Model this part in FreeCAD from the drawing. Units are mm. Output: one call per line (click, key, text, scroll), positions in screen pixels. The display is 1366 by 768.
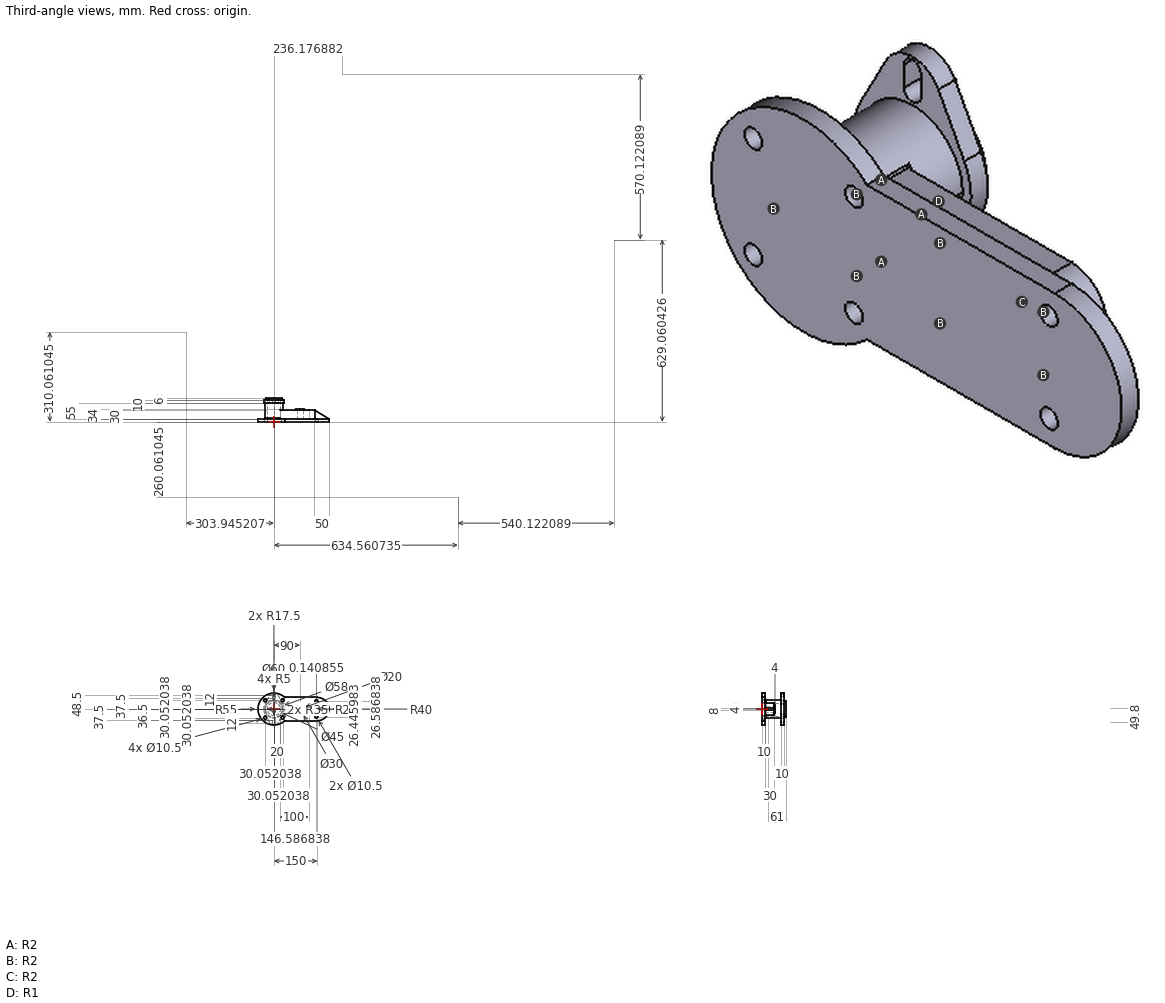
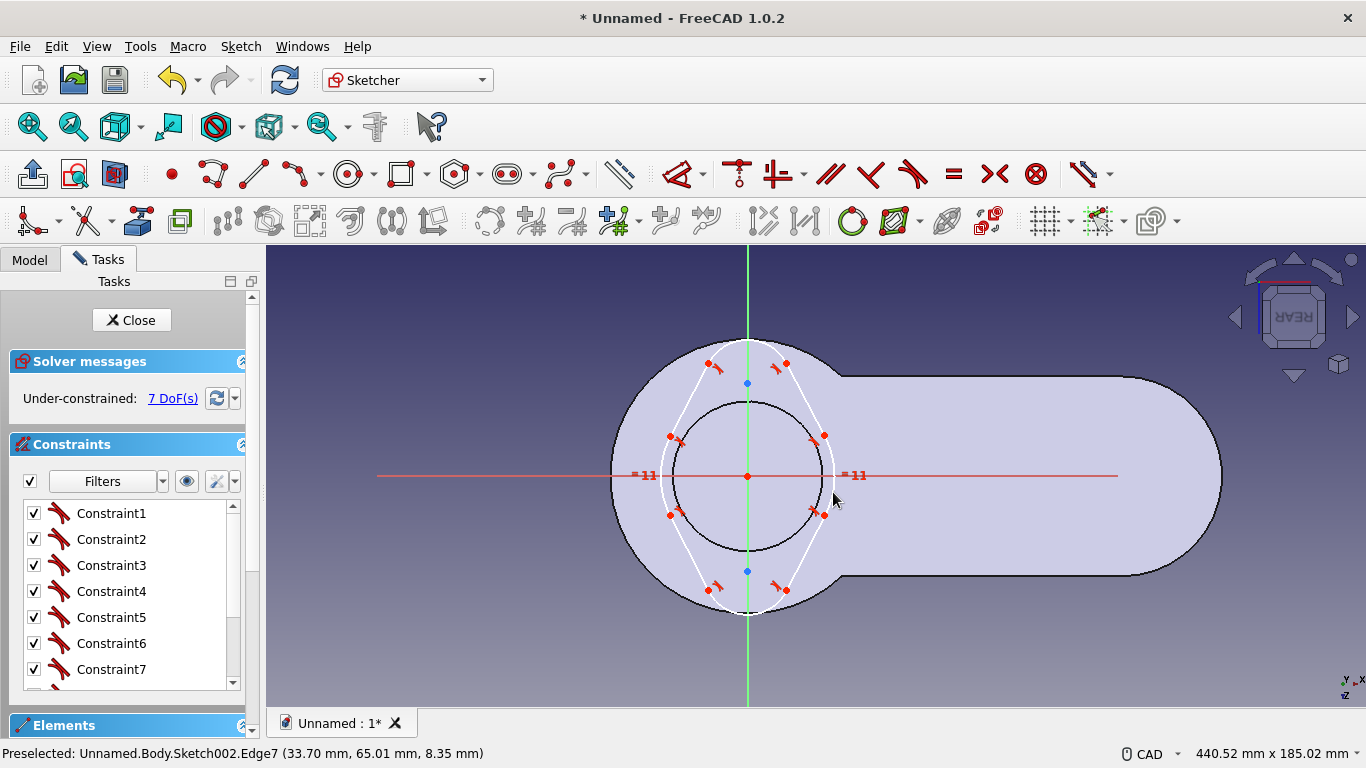
click(729, 611)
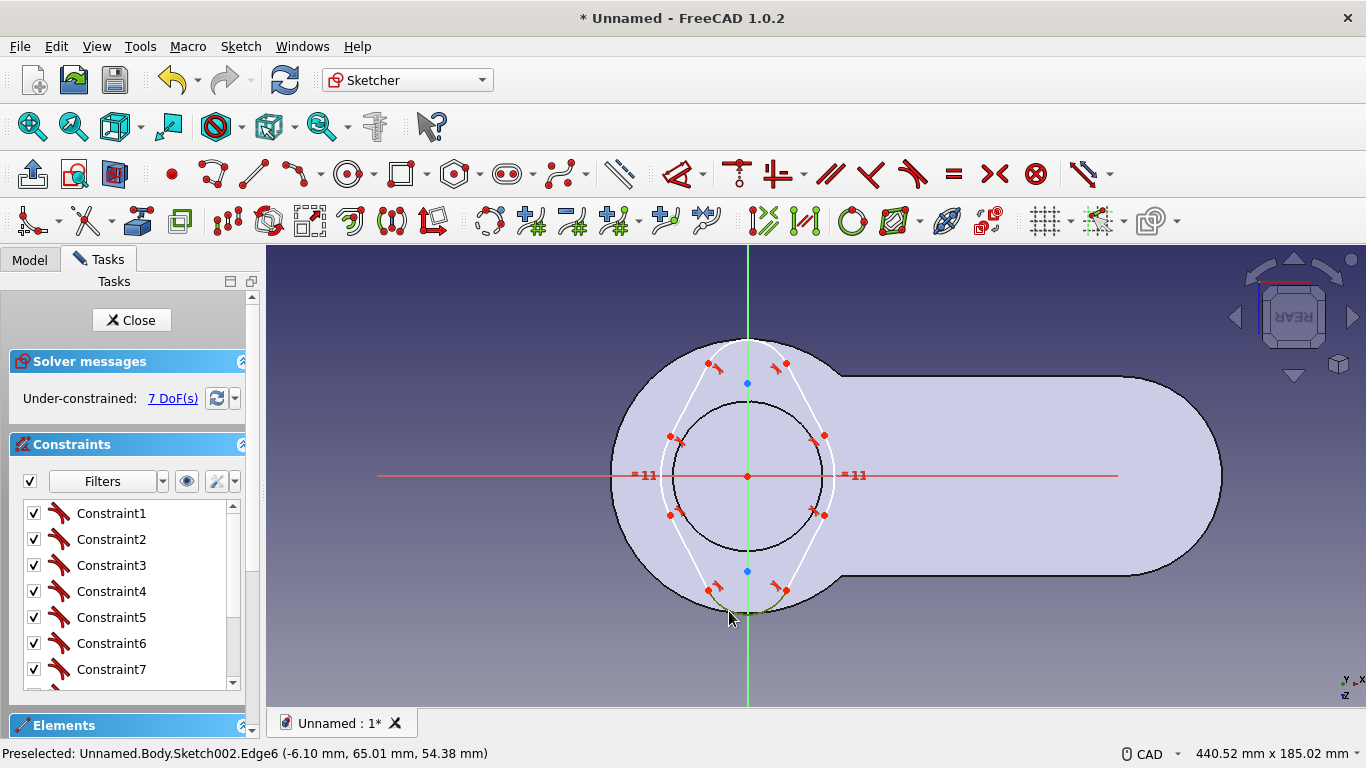
click(766, 344)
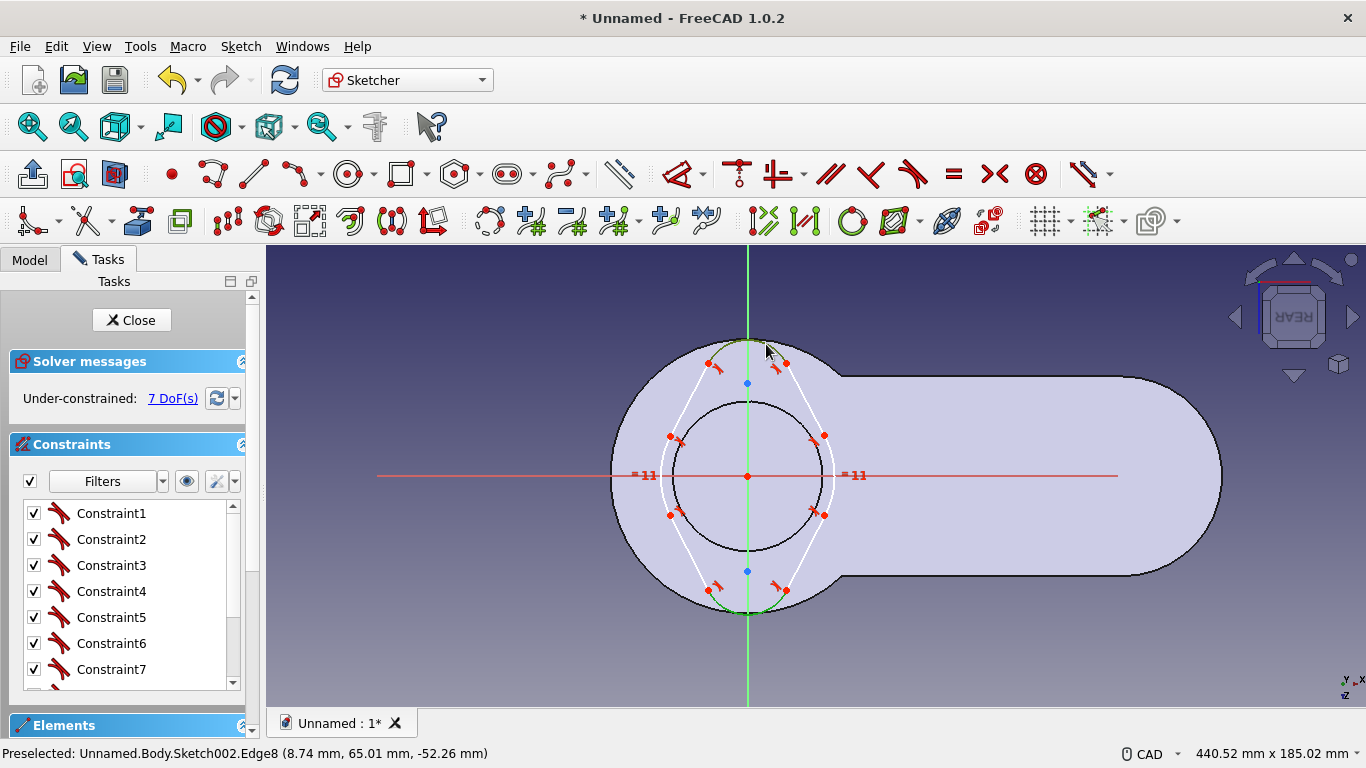
click(954, 174)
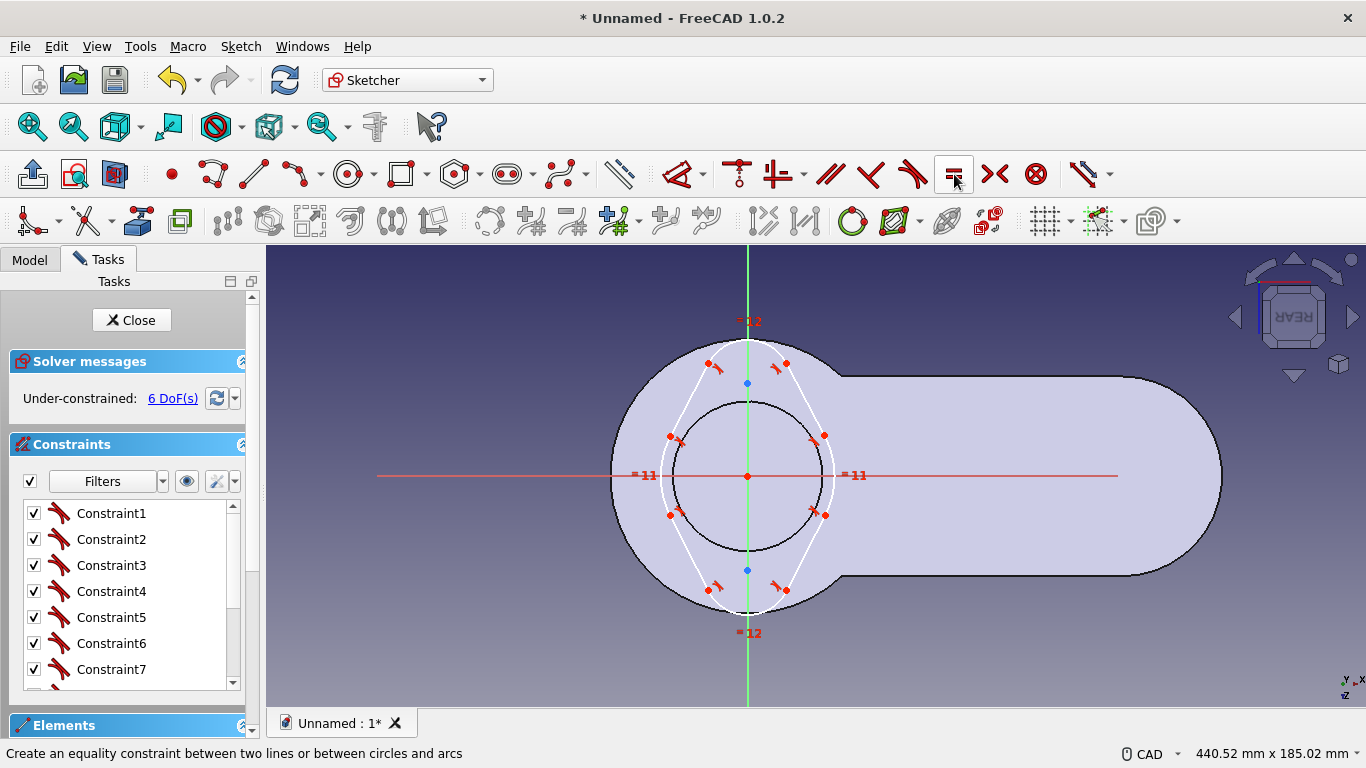
click(748, 571)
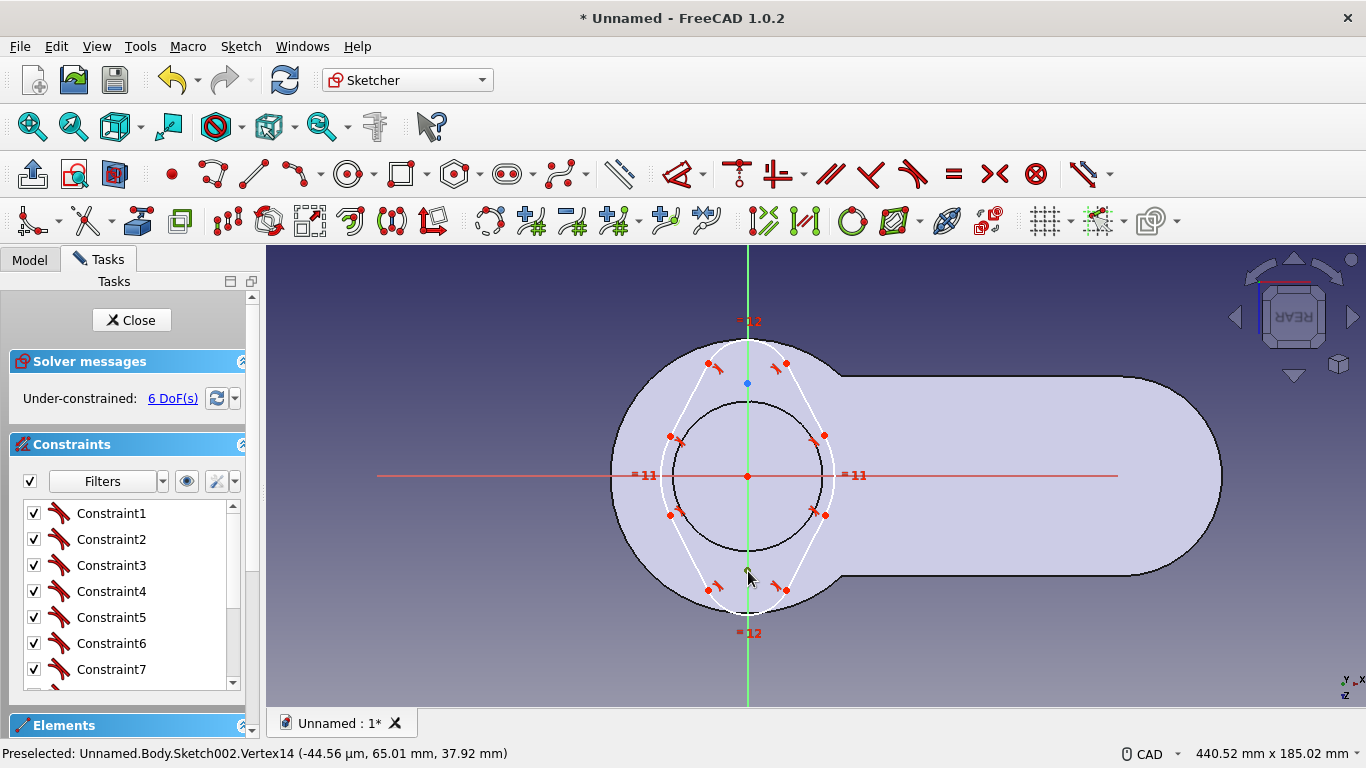
click(748, 650)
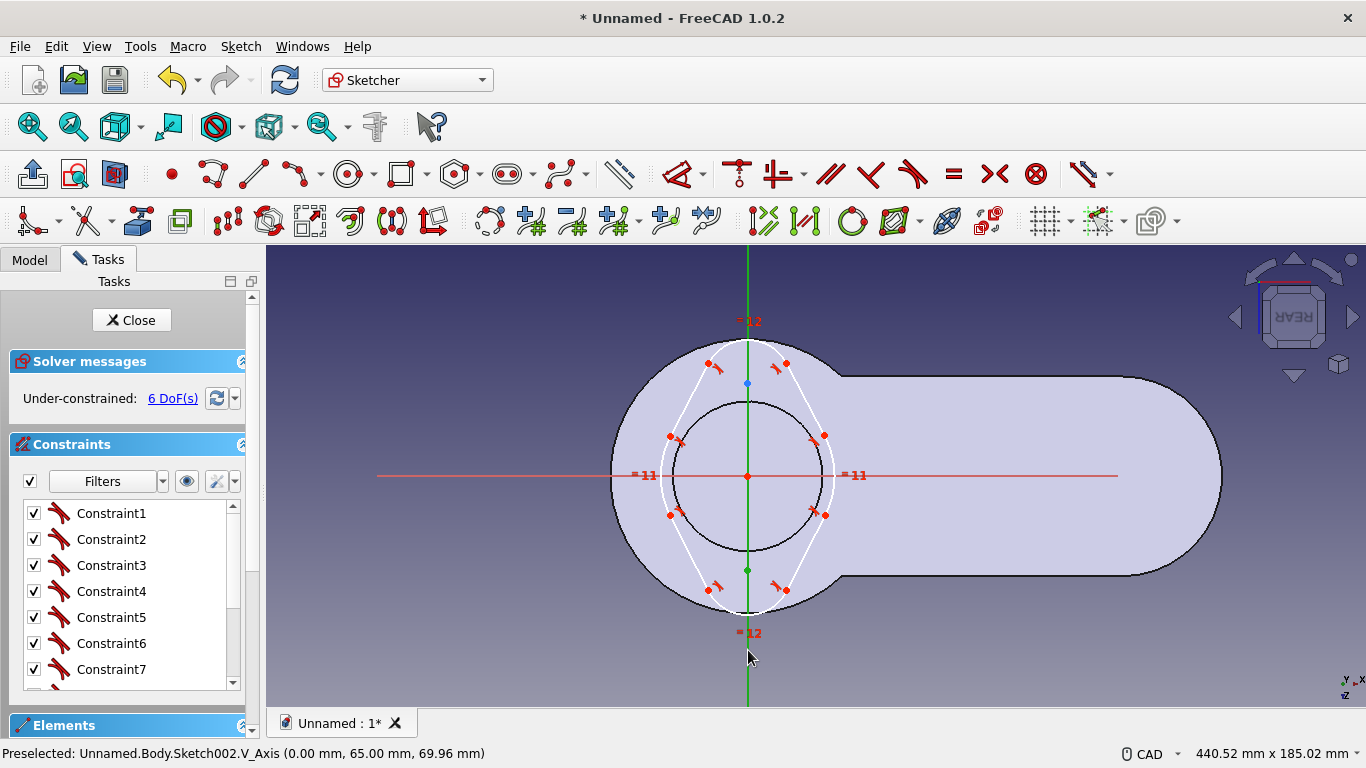
click(737, 174)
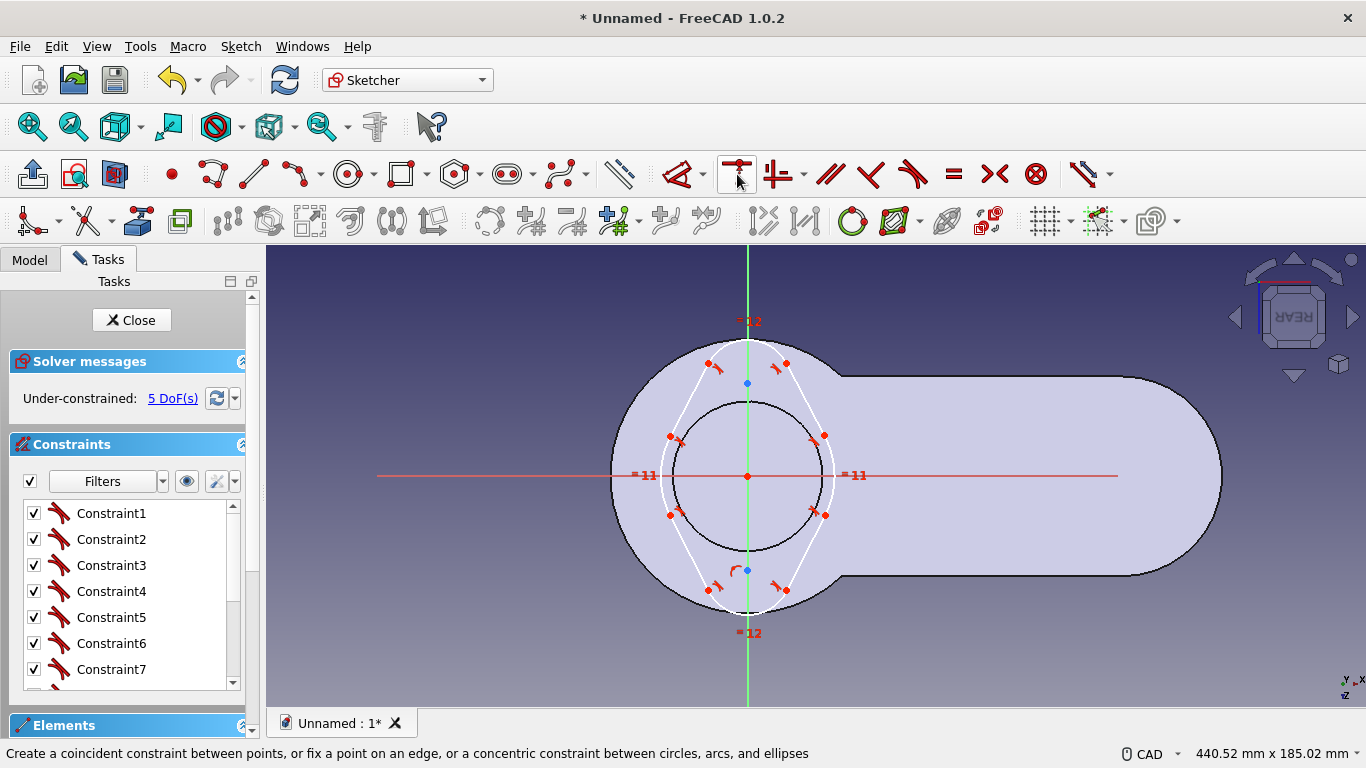
click(748, 384)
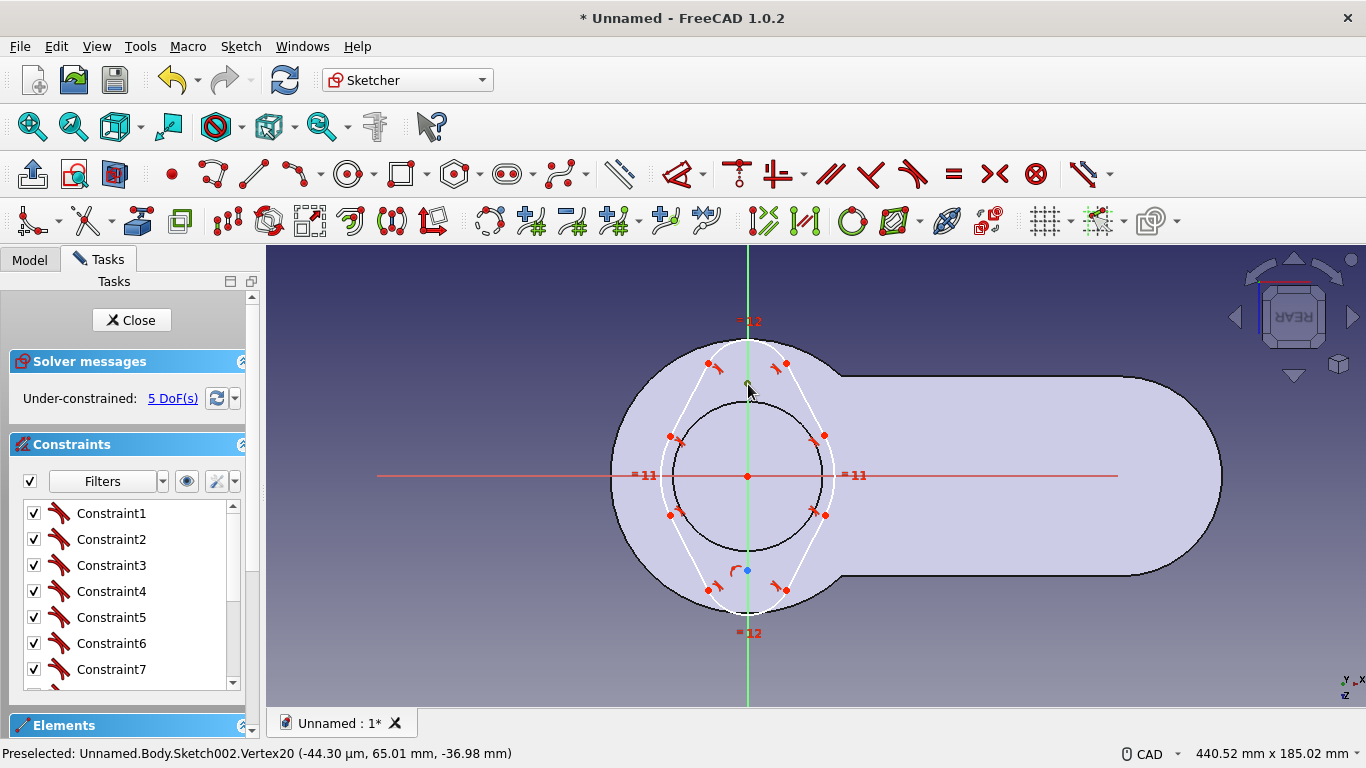
click(748, 650)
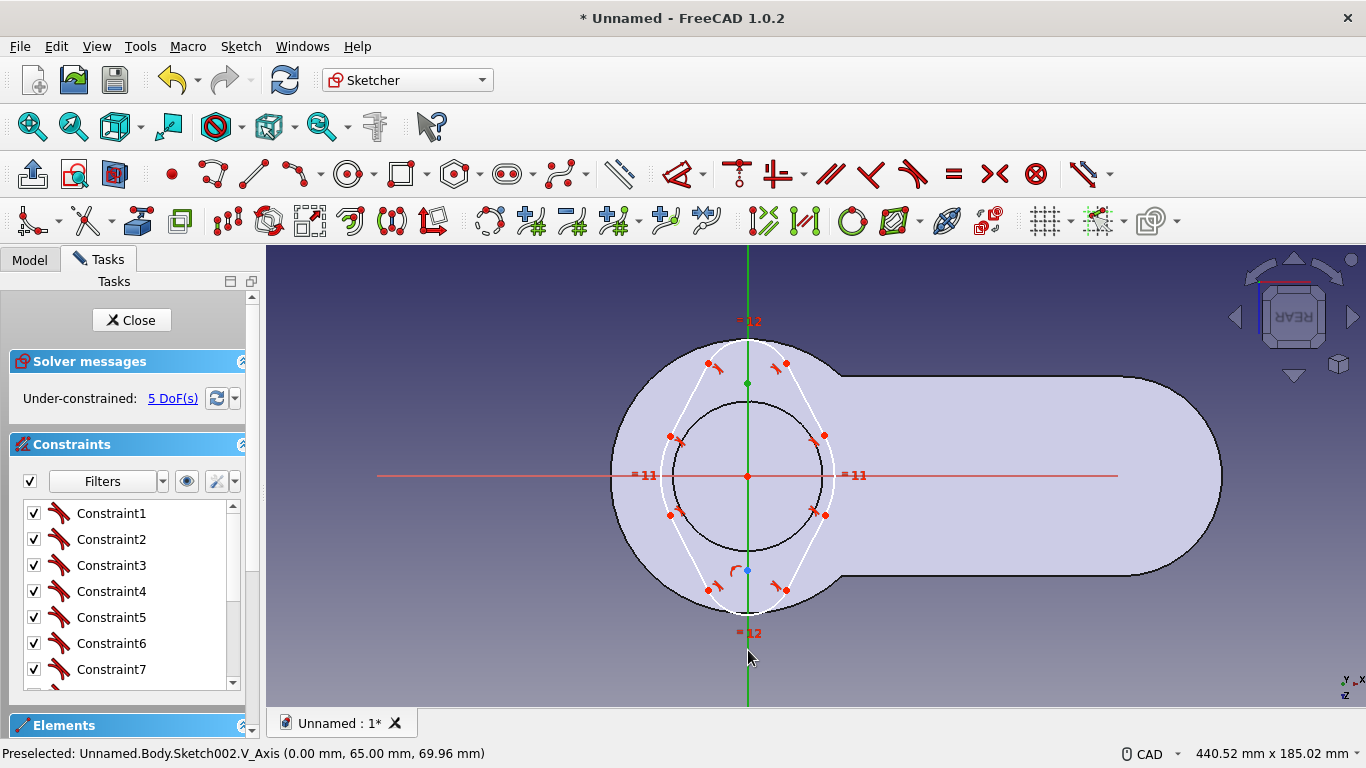
key(c)